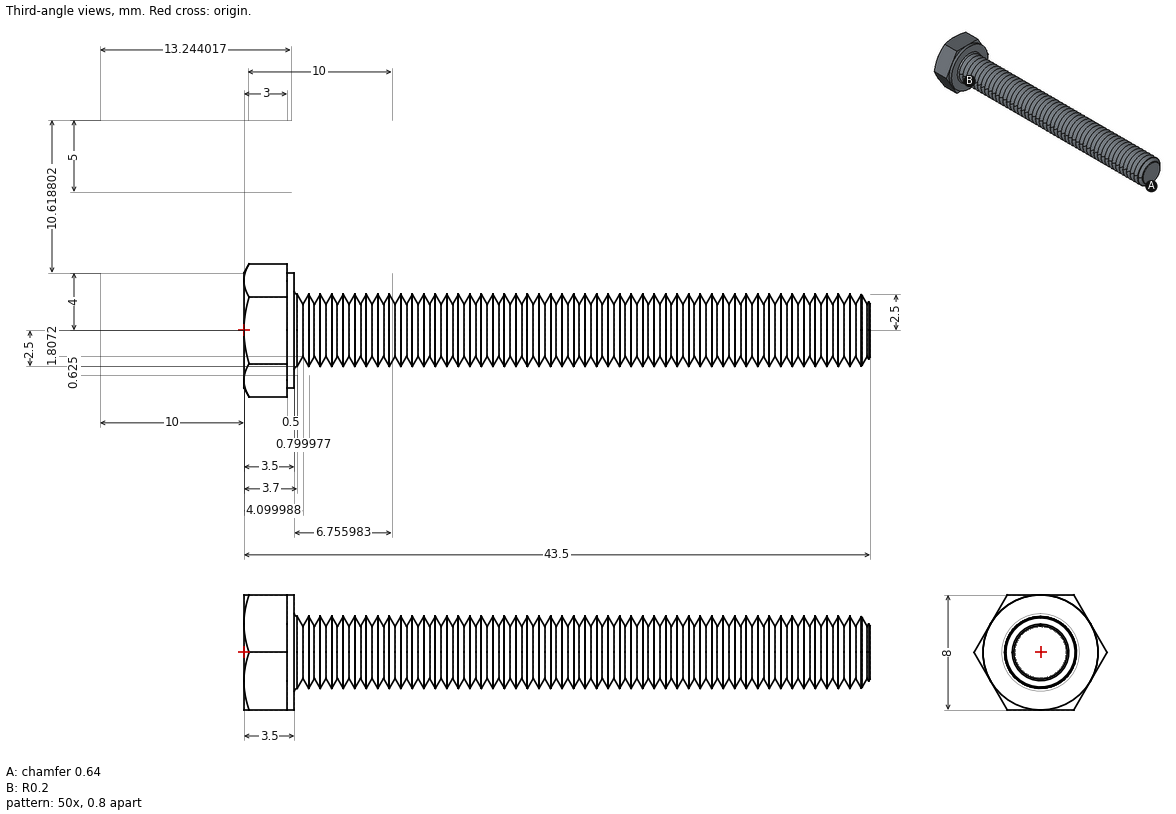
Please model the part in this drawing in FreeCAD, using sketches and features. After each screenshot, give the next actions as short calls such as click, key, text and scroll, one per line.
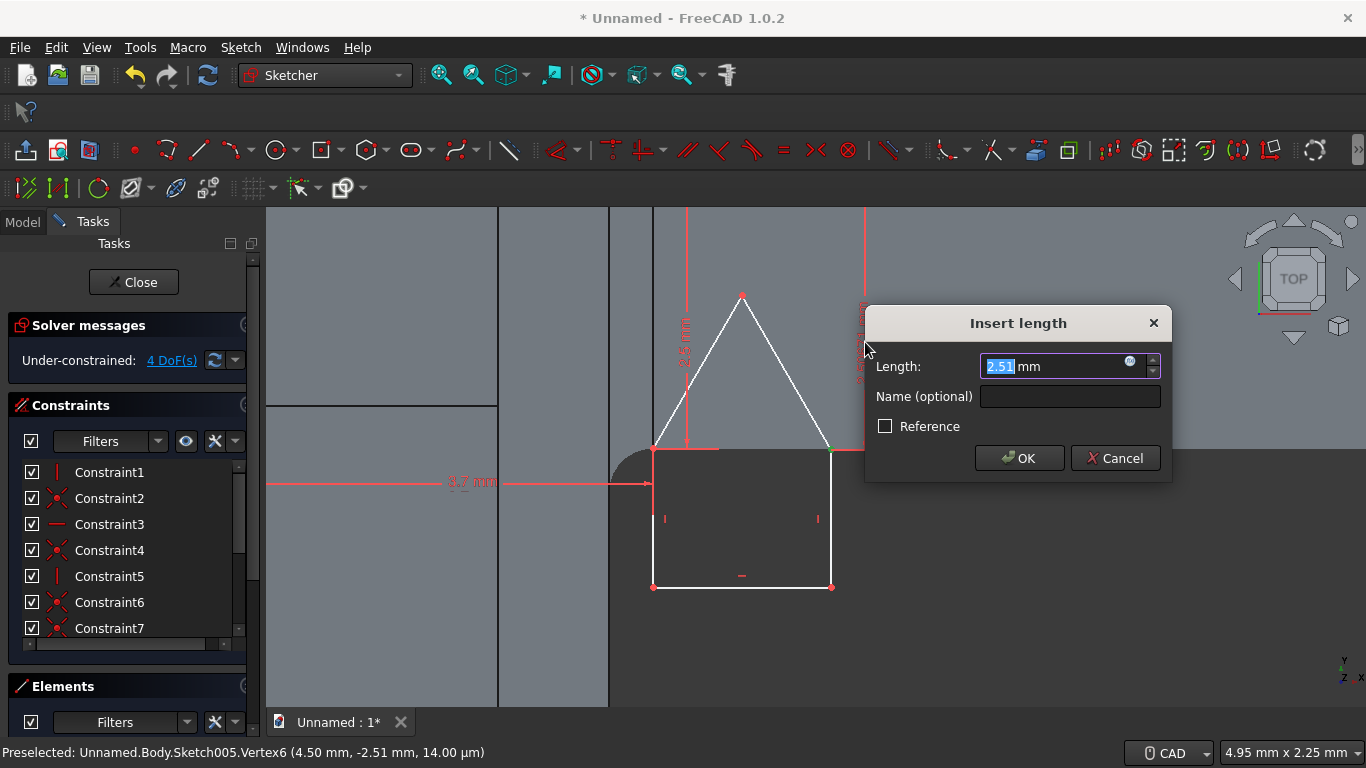
text(2.5)
key(Return)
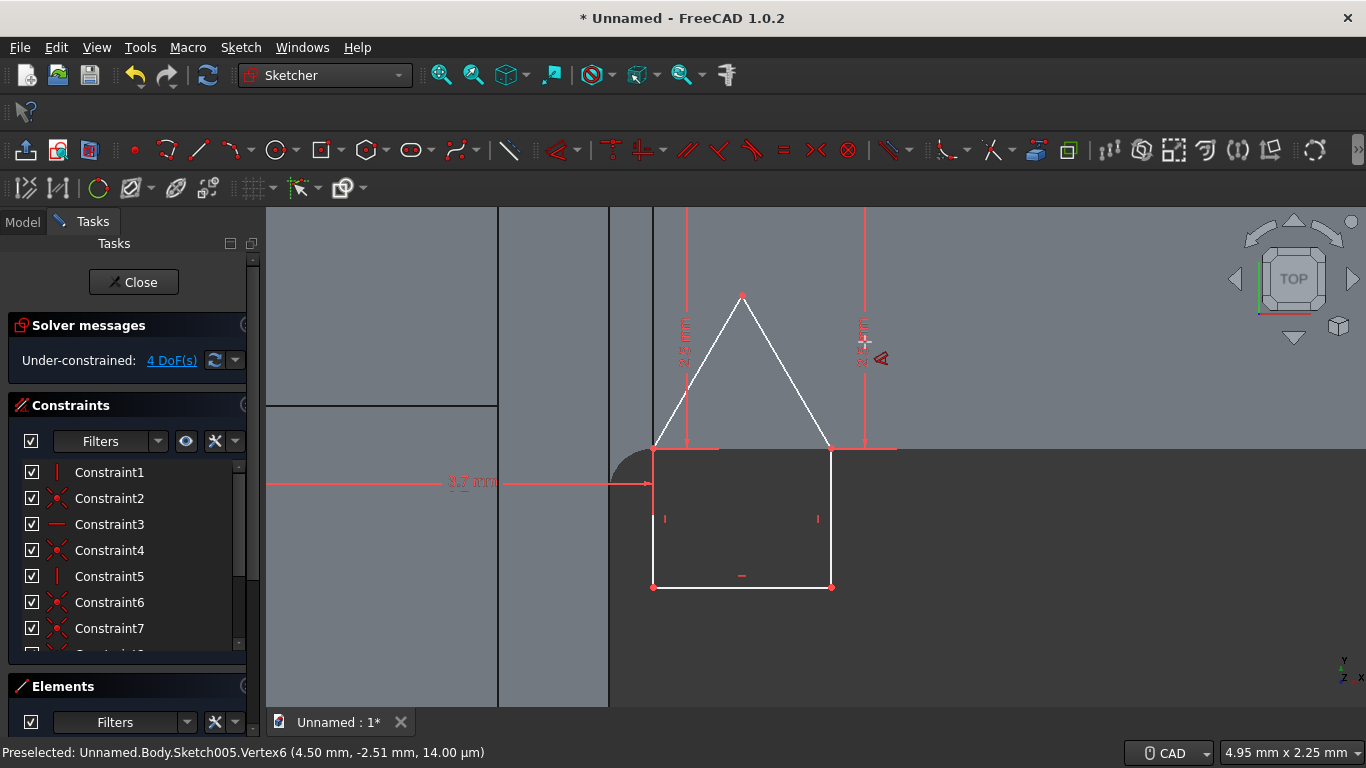
click(653, 490)
click(619, 518)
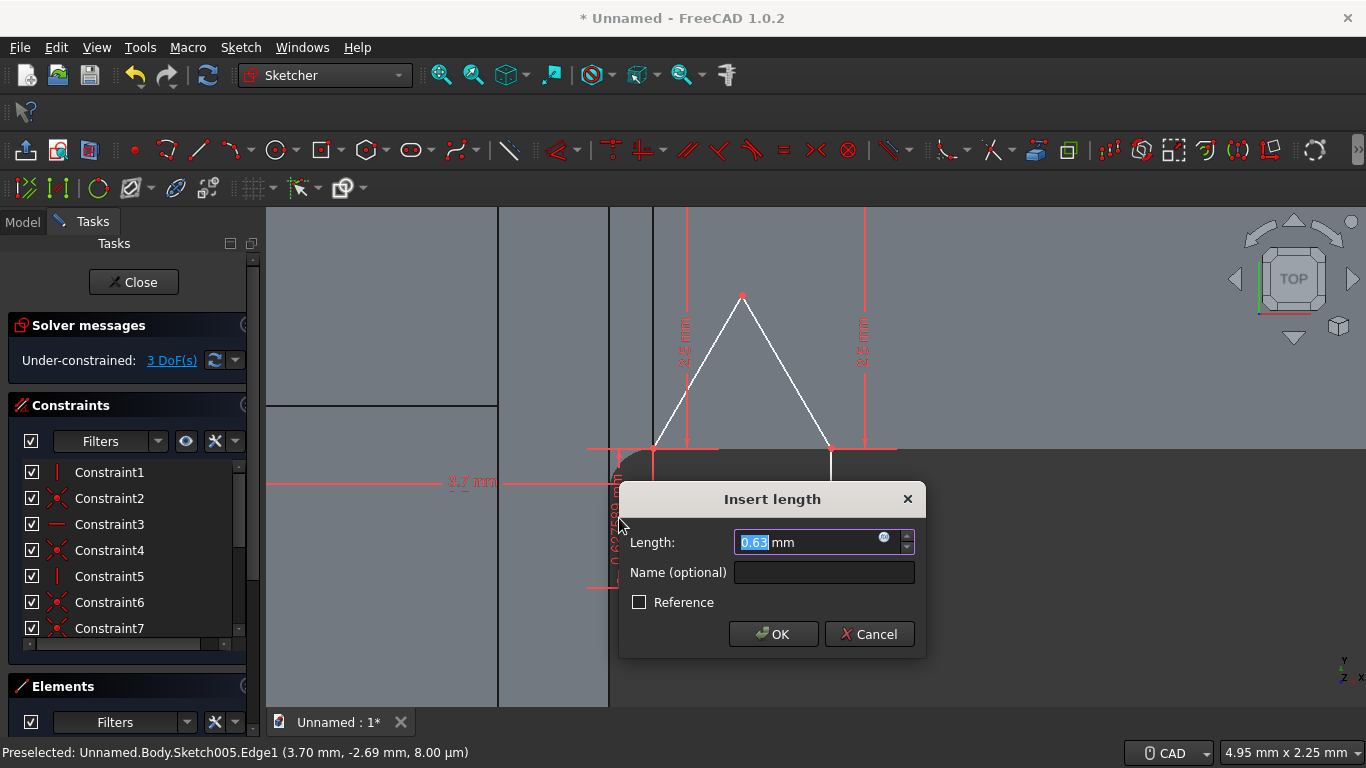
text(0.625)
key(Return)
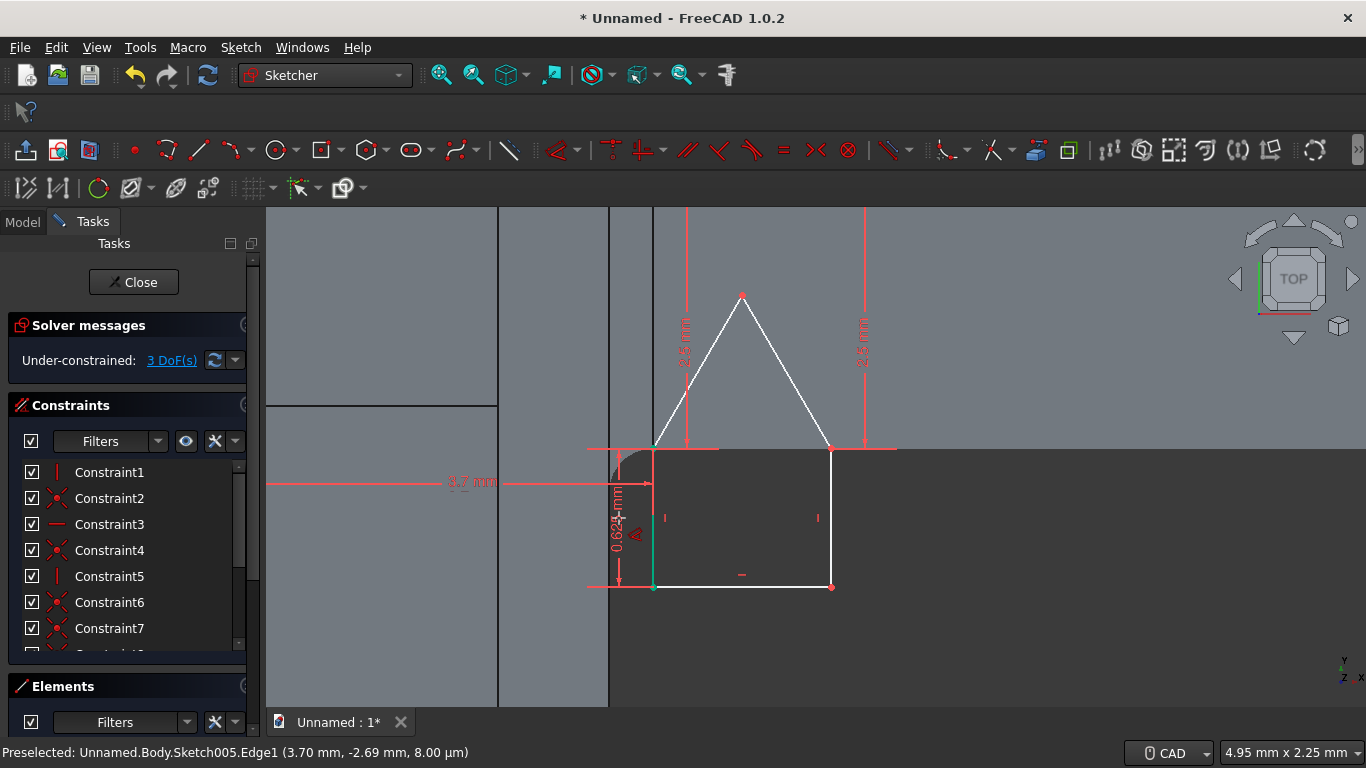
click(742, 296)
click(776, 266)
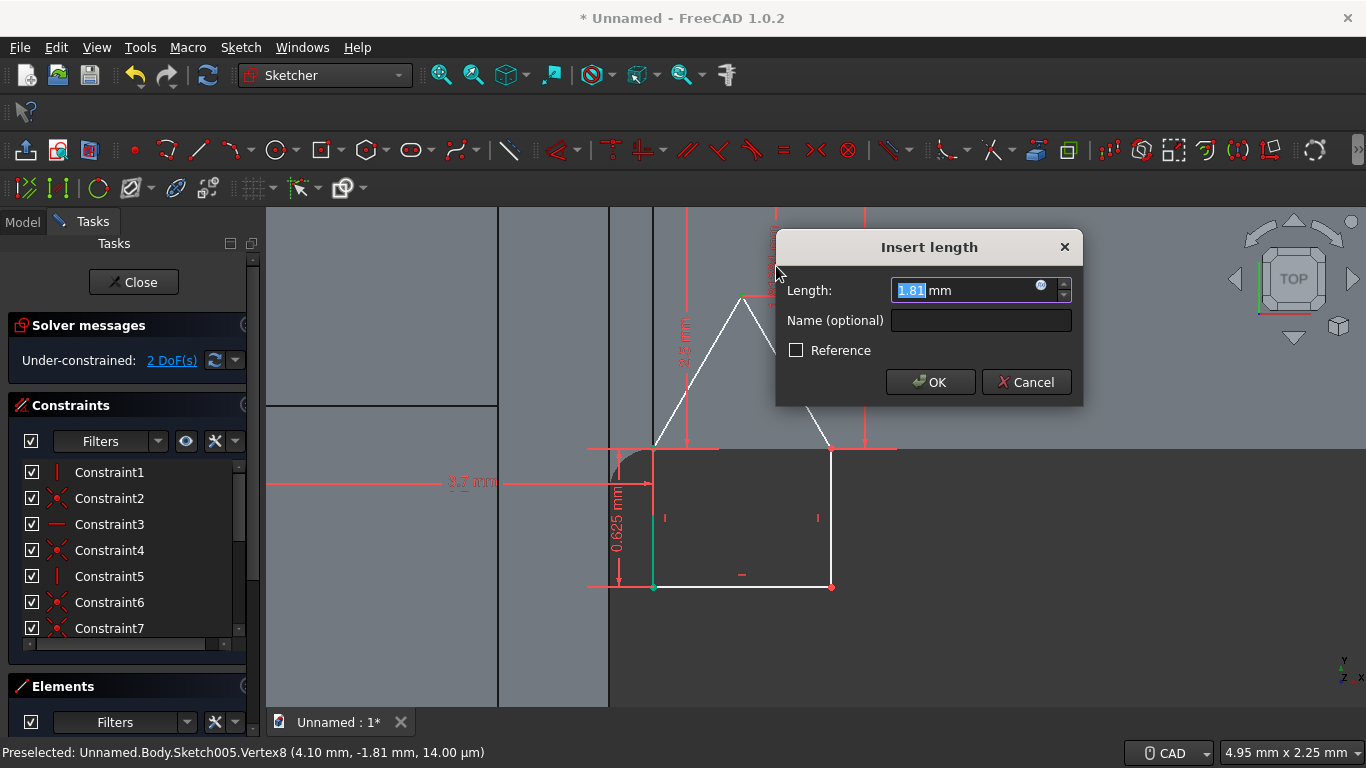
text(1.8072)
key(Return)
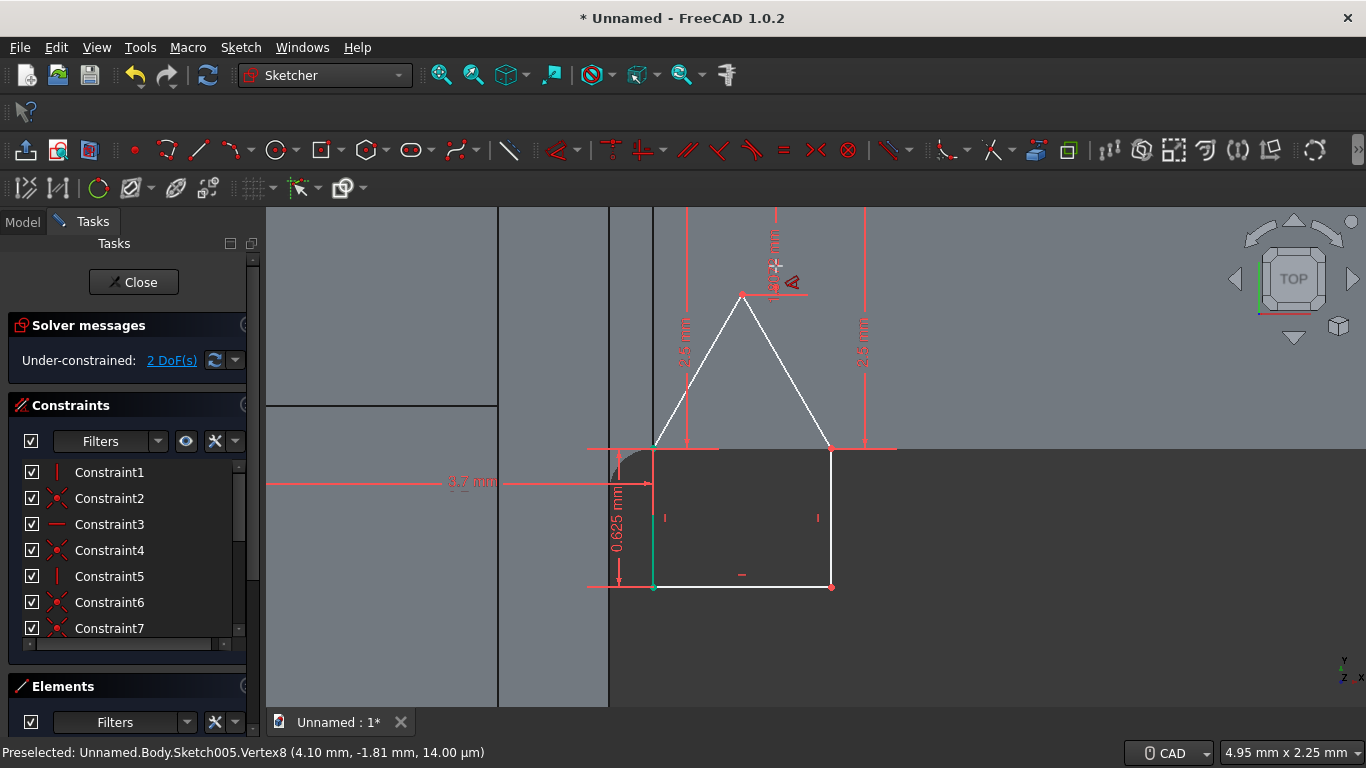
click(707, 587)
click(742, 621)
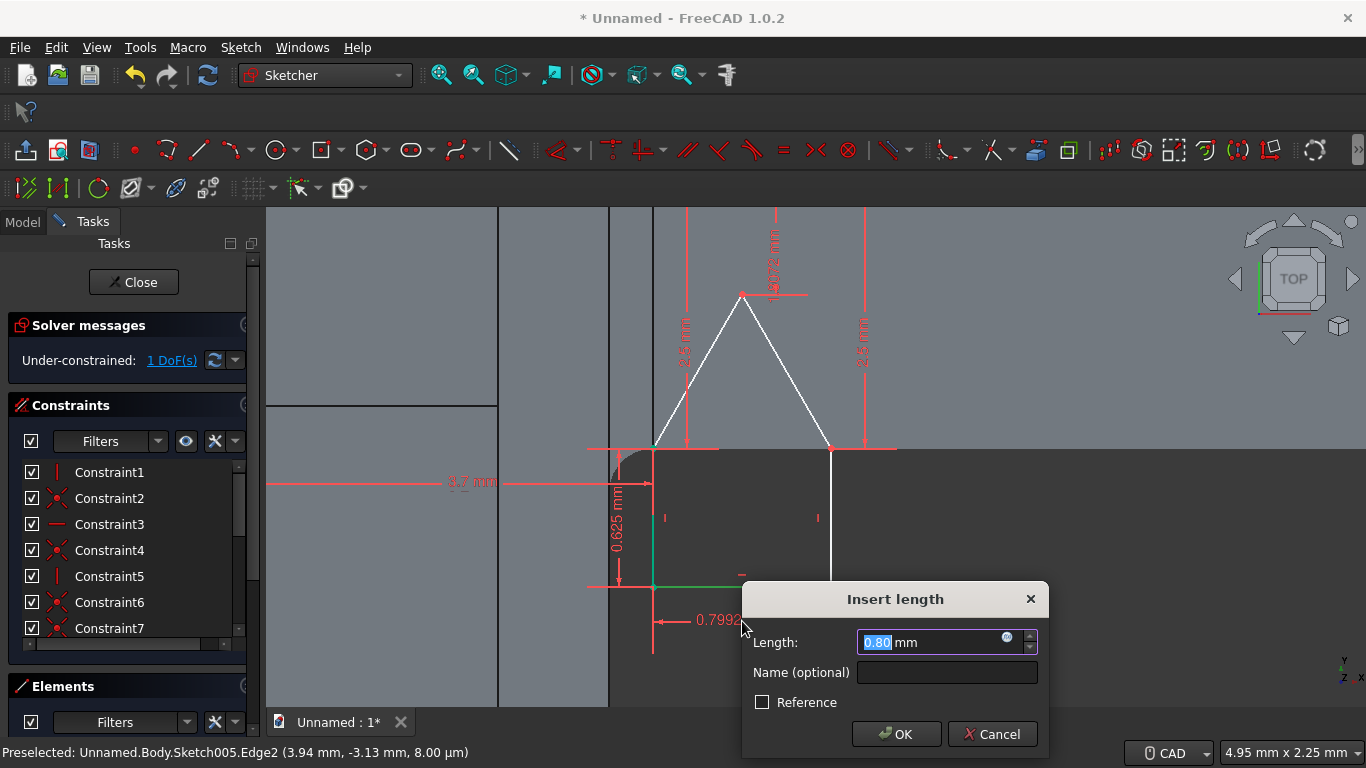
text(0.799977)
key(Return)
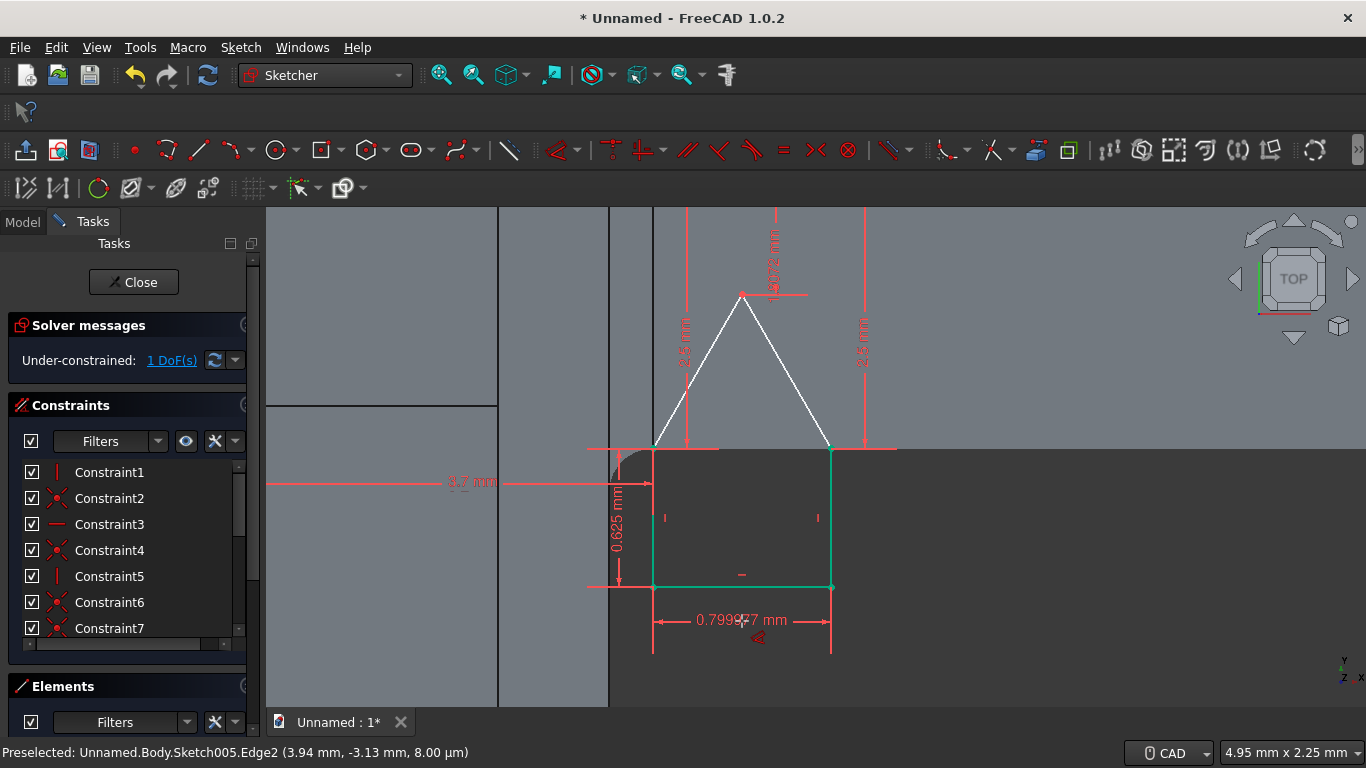
click(742, 295)
click(518, 329)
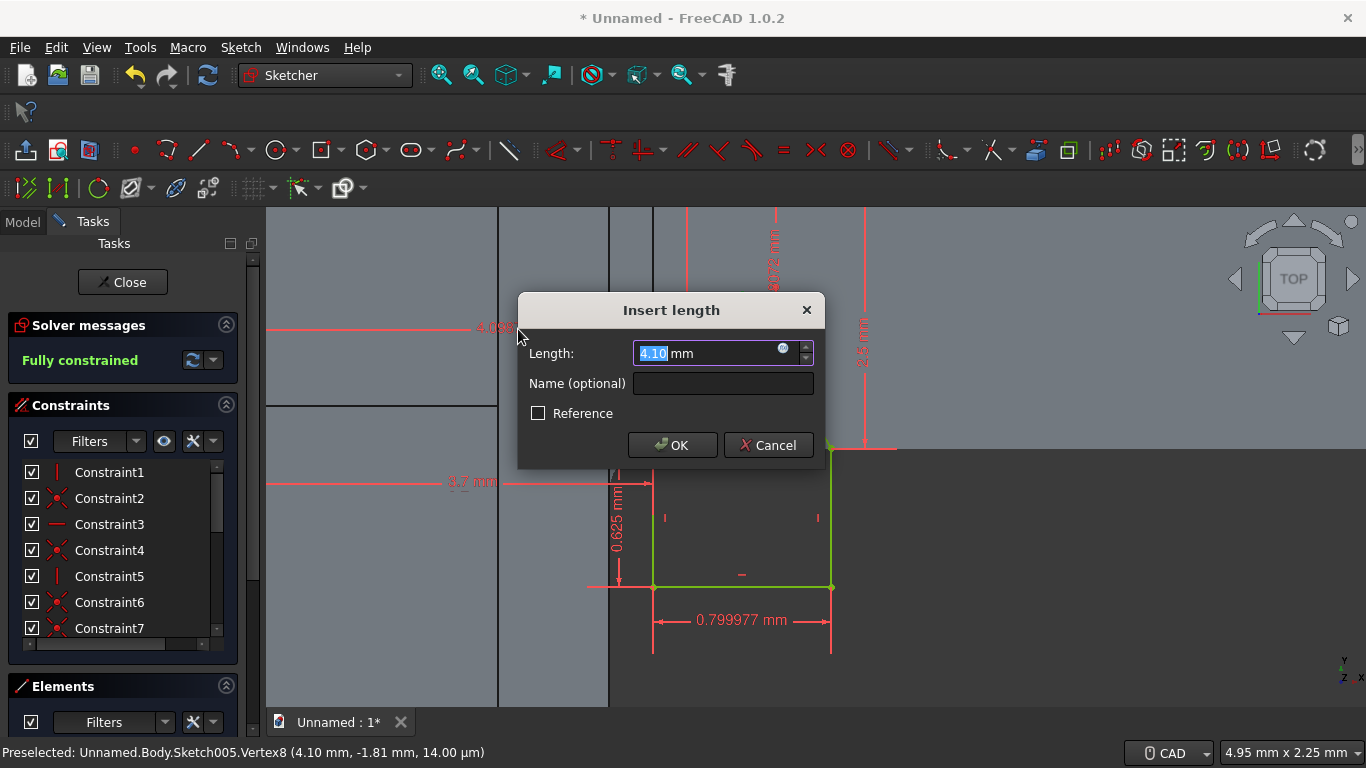
text(4.099988)
key(Return)
key(Escape)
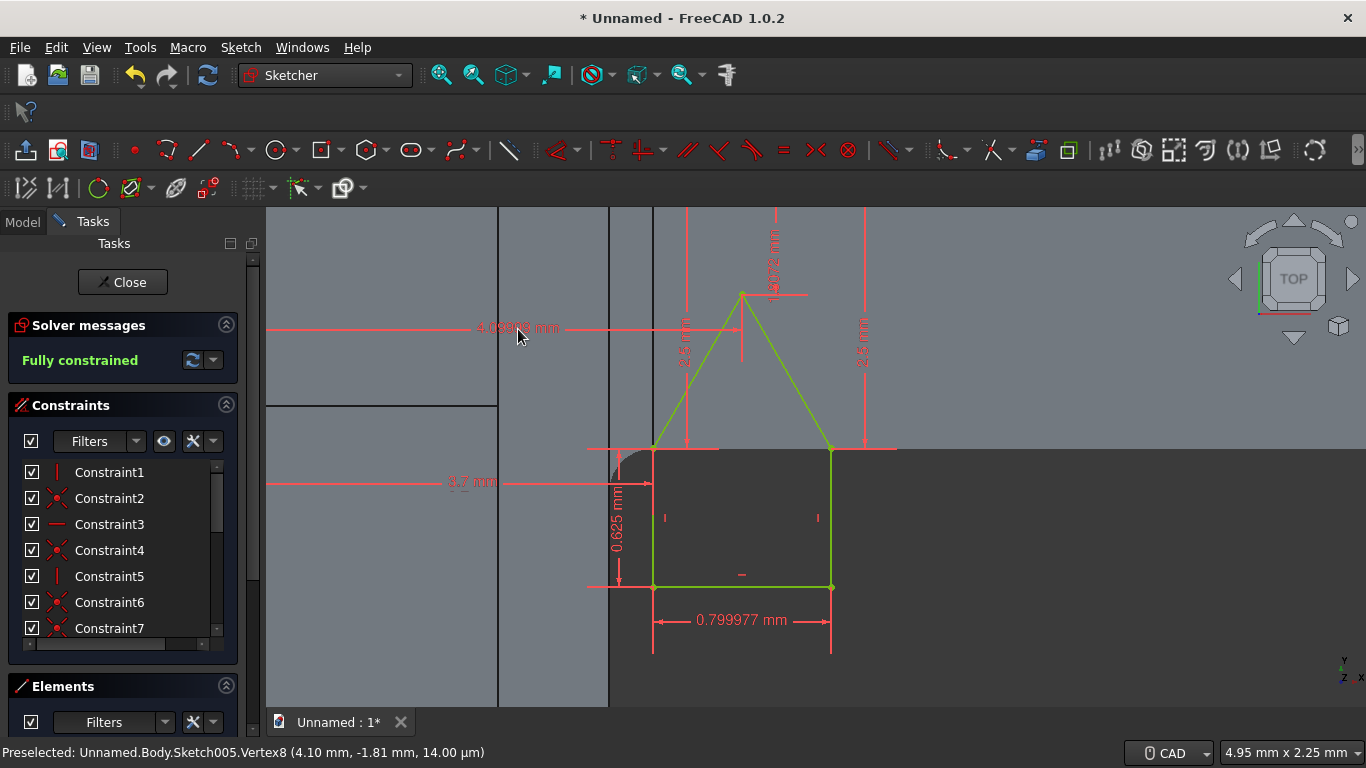
click(123, 282)